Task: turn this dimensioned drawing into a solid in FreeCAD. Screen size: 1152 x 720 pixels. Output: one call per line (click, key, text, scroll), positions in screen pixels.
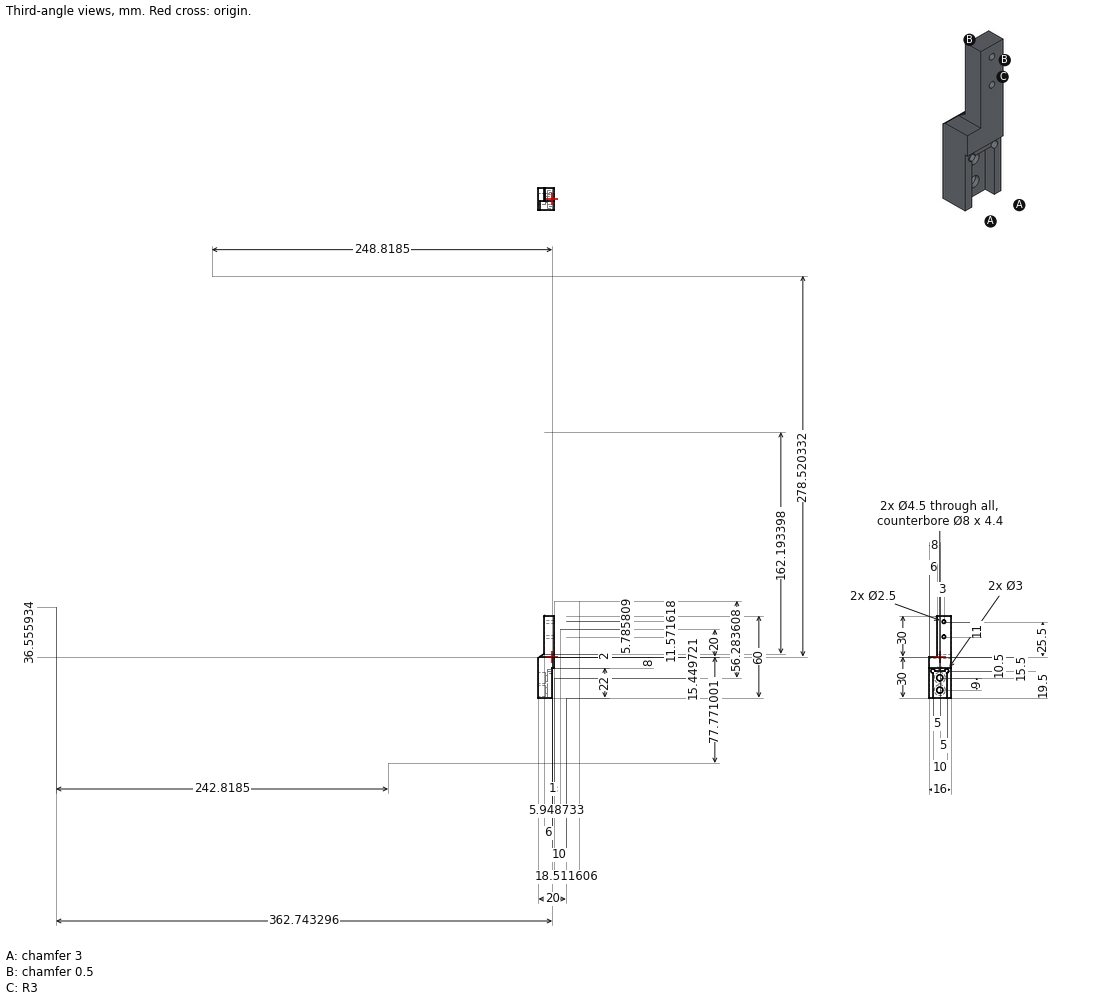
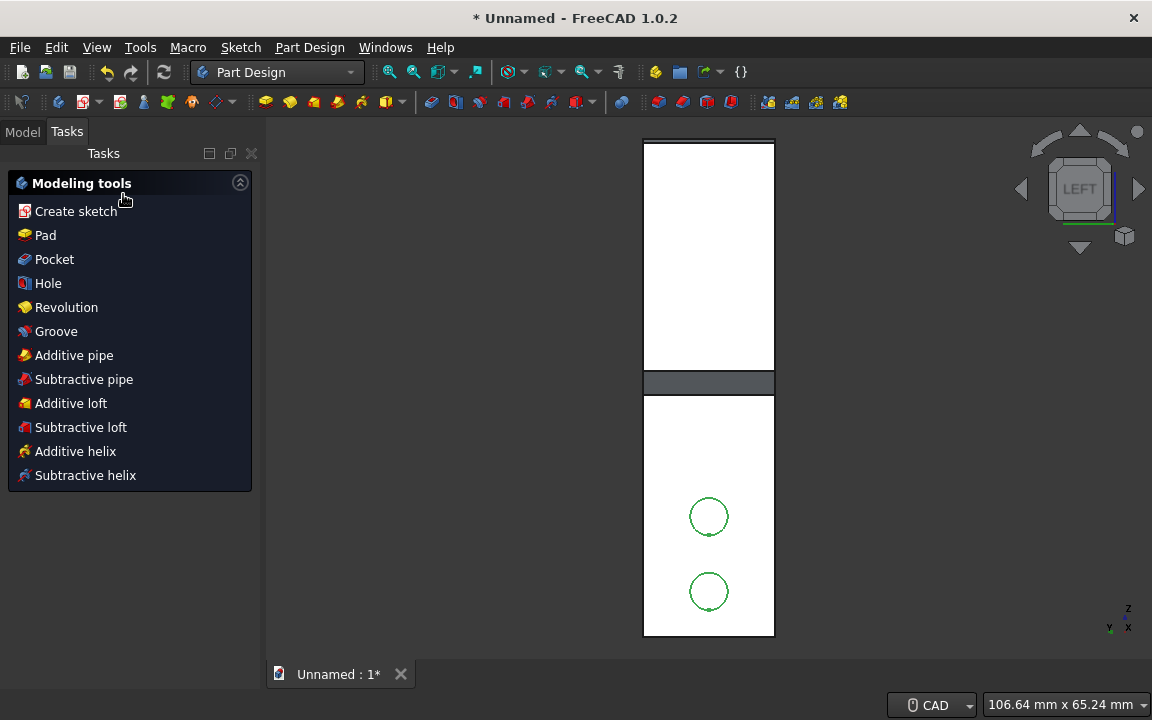
click(456, 102)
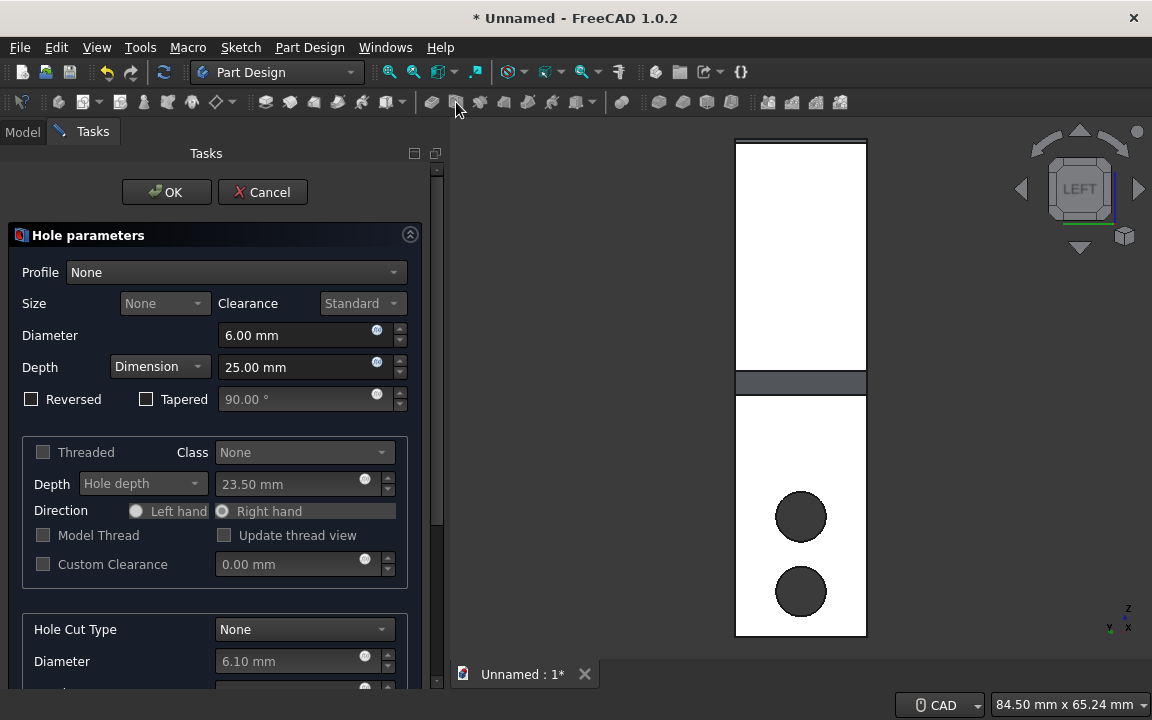
triple_click(305, 335)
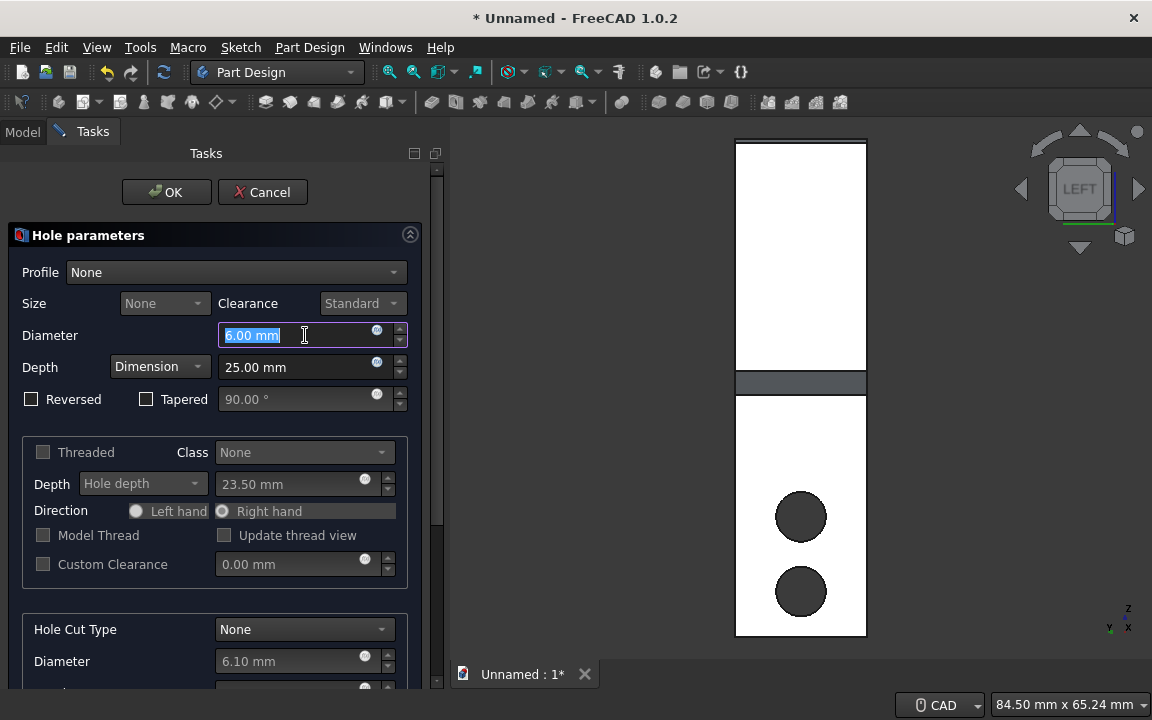
text(4.5)
key(Tab)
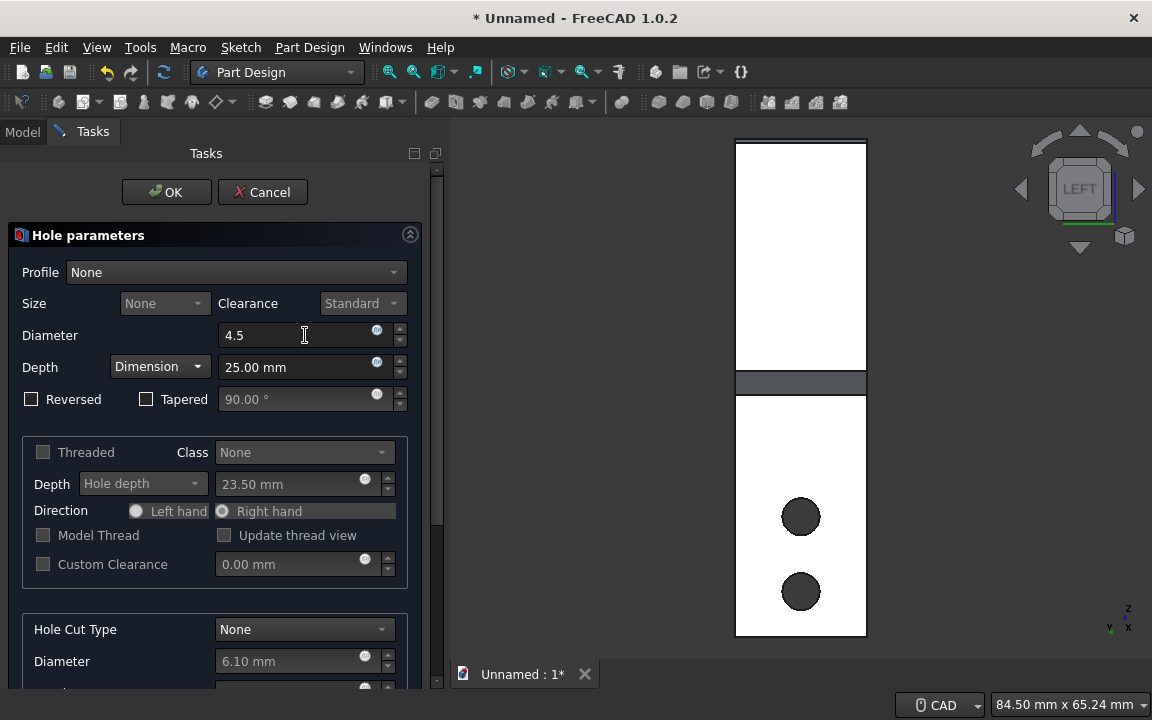
click(161, 366)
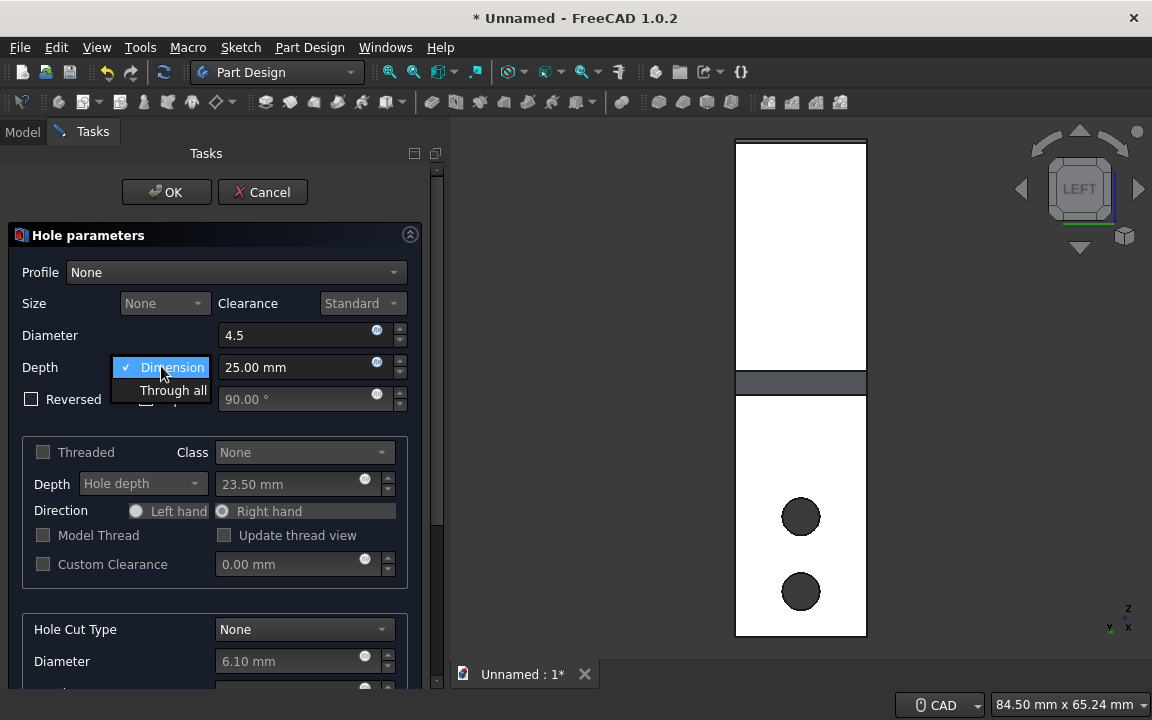
click(160, 390)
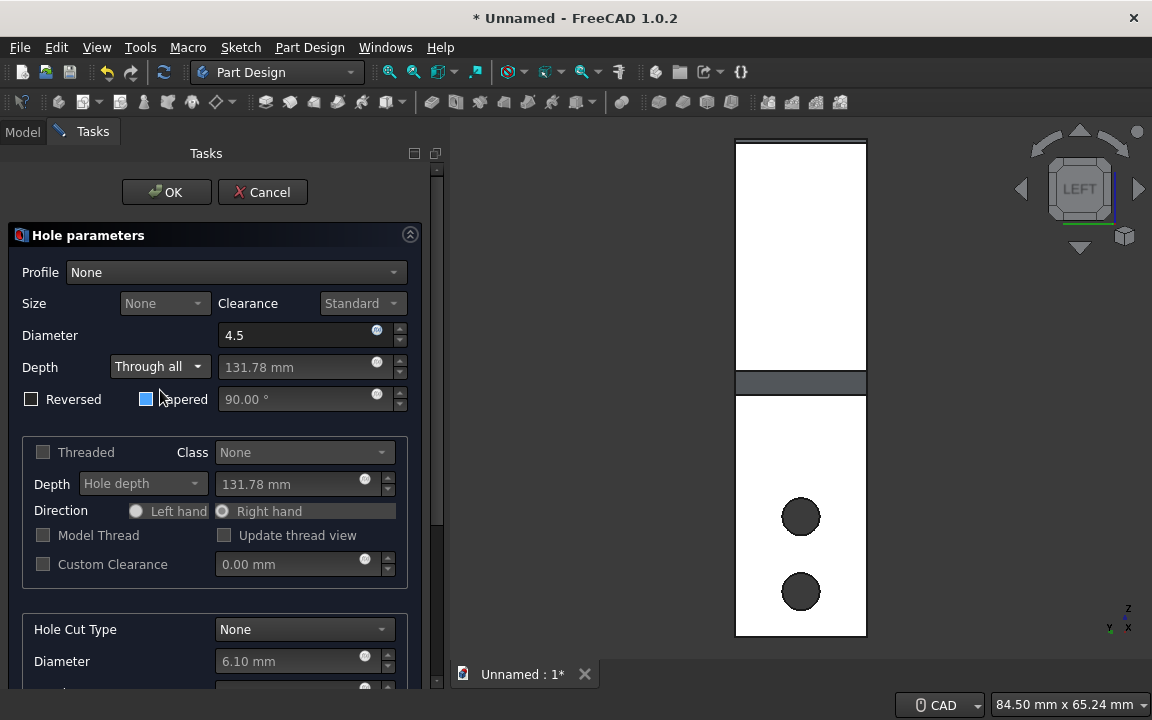
click(306, 630)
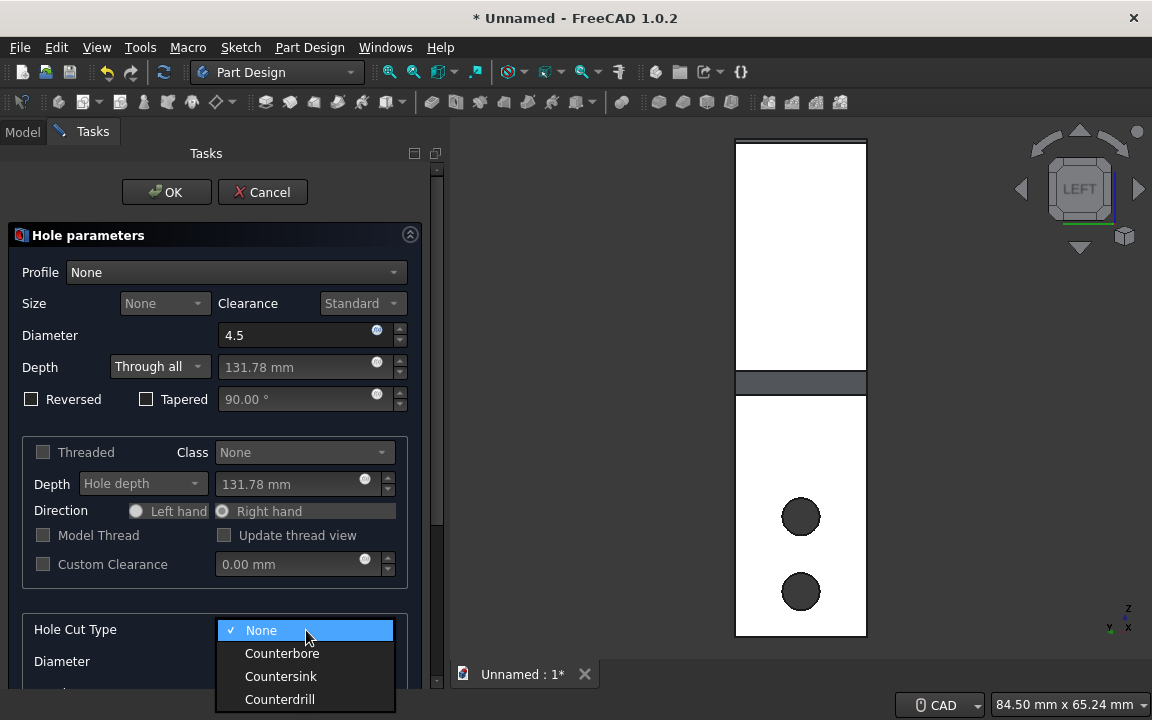
click(304, 654)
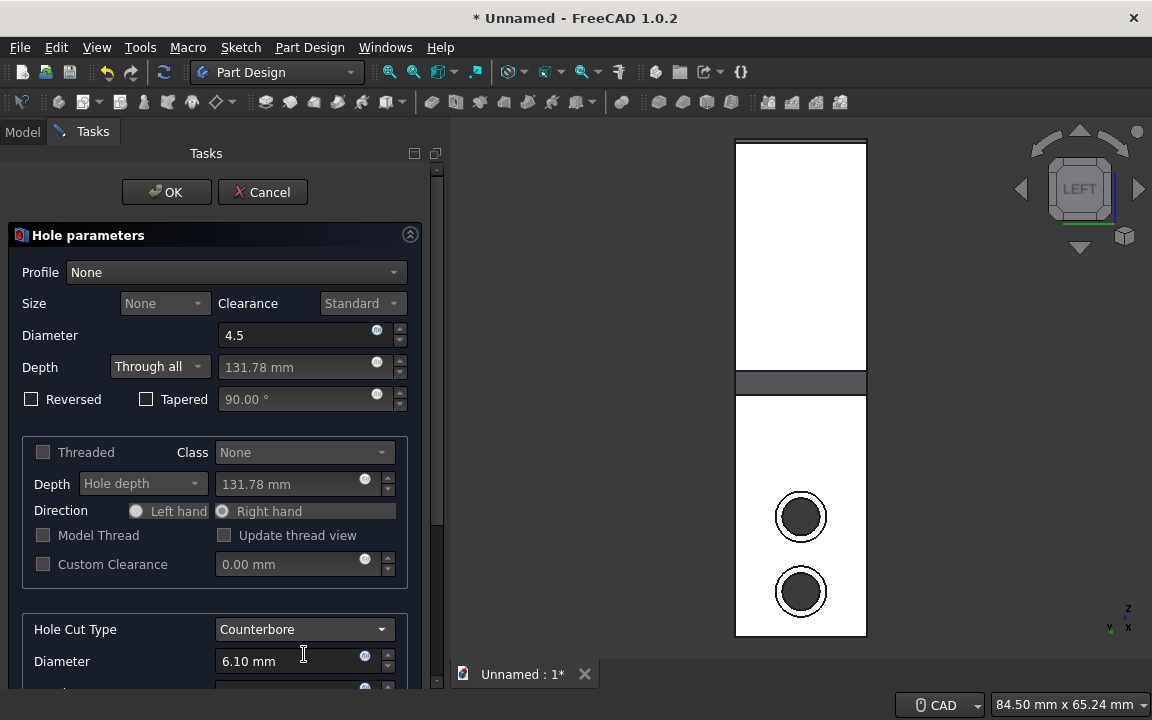
triple_click(298, 661)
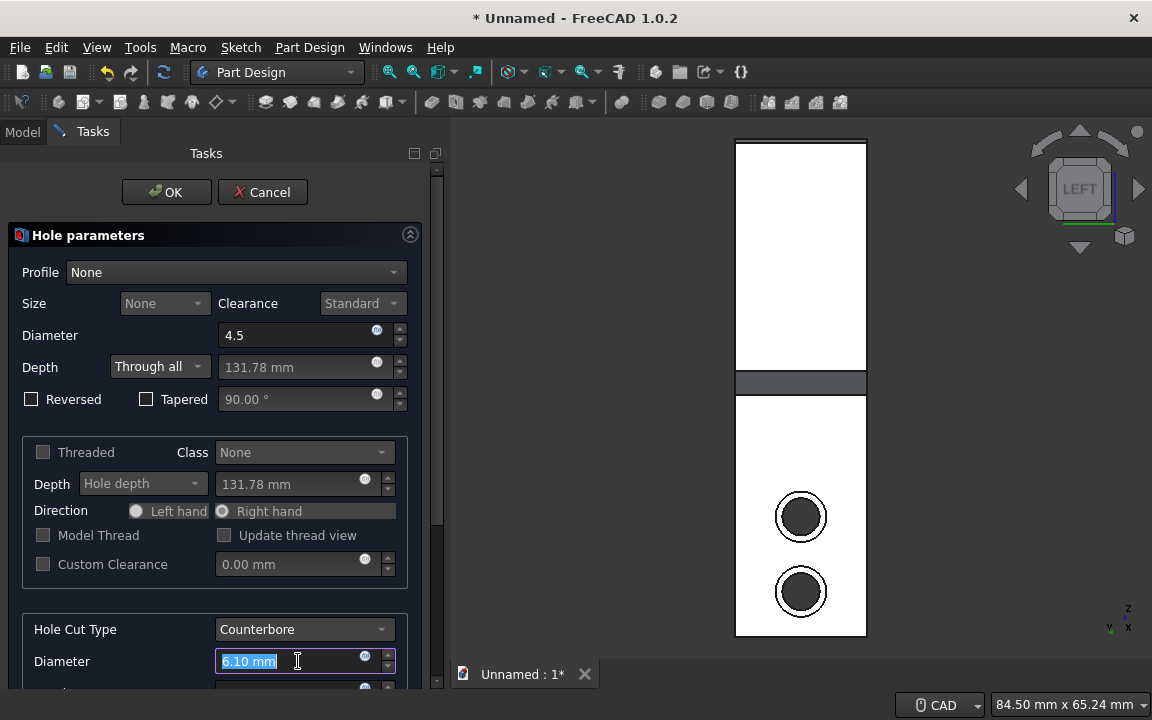
text(8)
key(Tab)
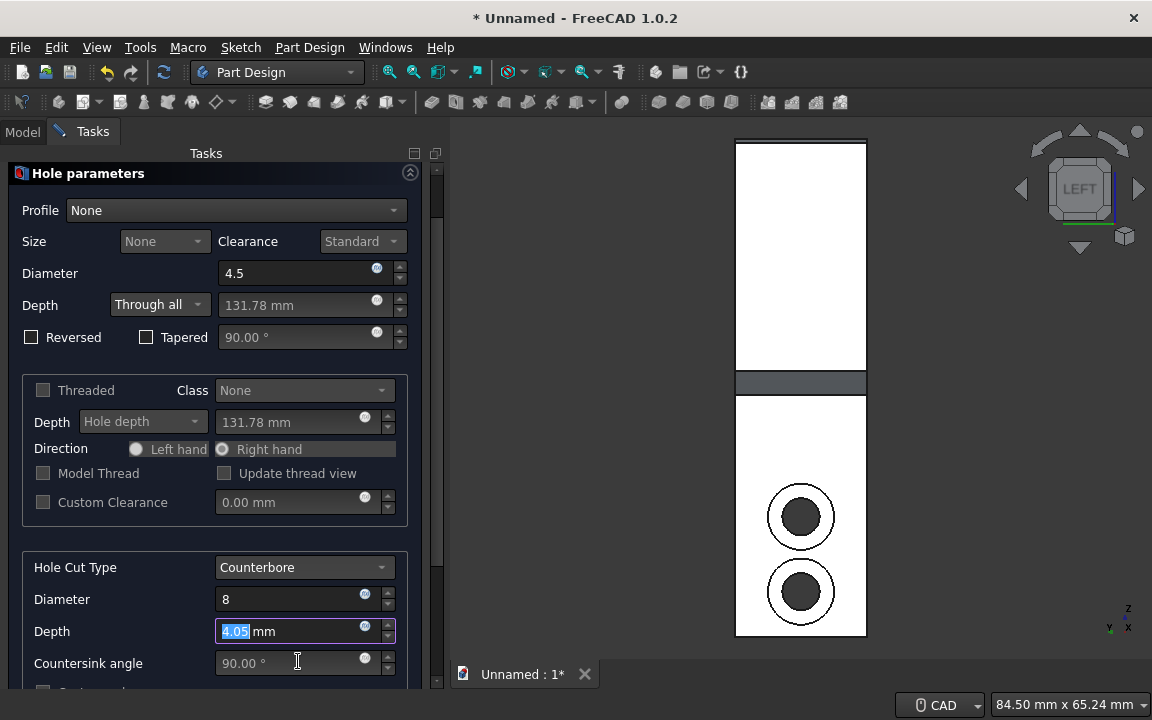
text(4.4)
key(Tab)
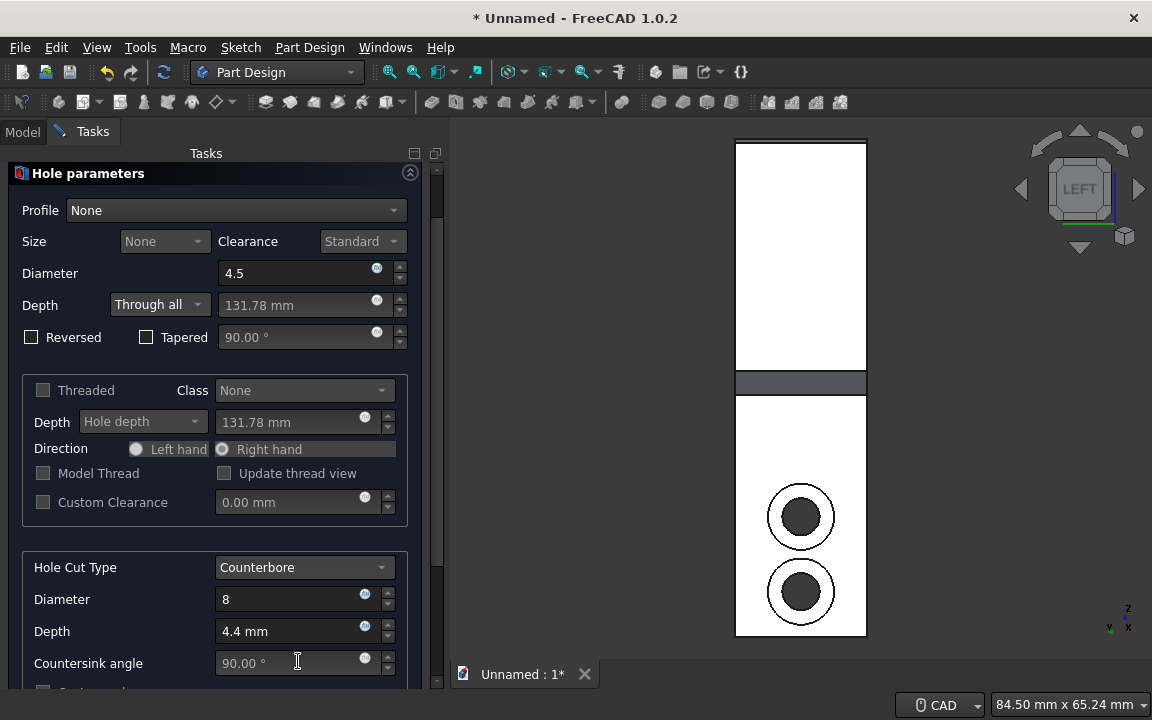
scroll(437, 426, up, 2)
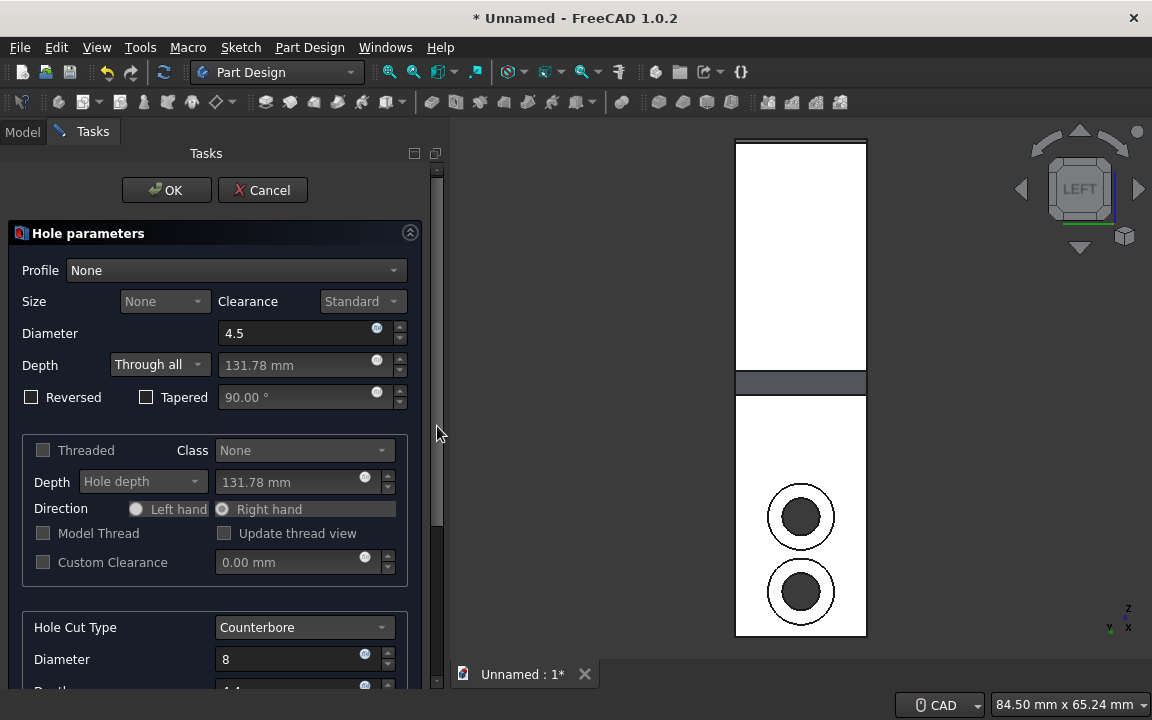
click(167, 192)